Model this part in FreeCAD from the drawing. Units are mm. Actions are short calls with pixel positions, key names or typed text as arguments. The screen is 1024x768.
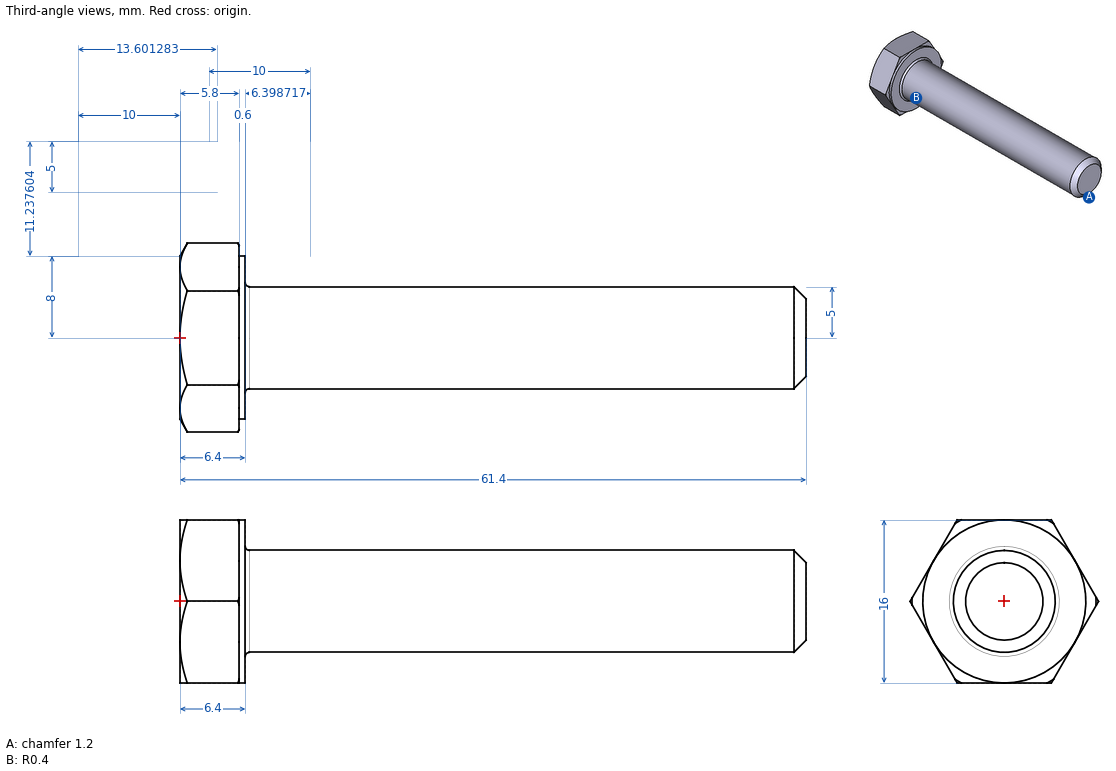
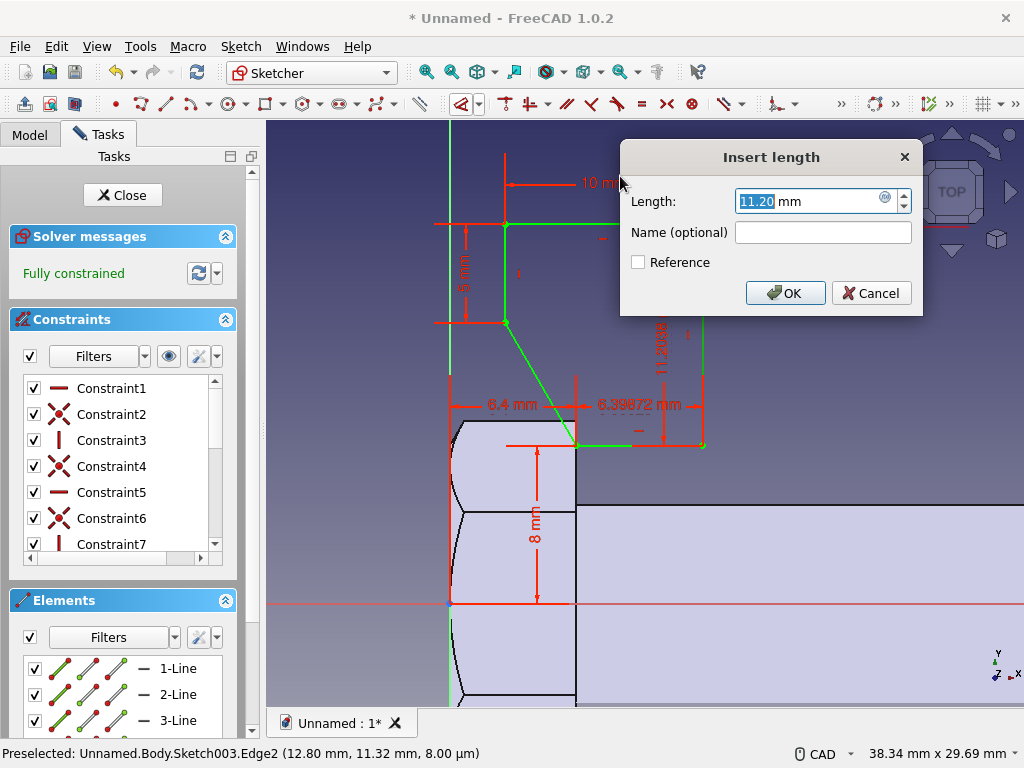
text(11.237604)
key(Return)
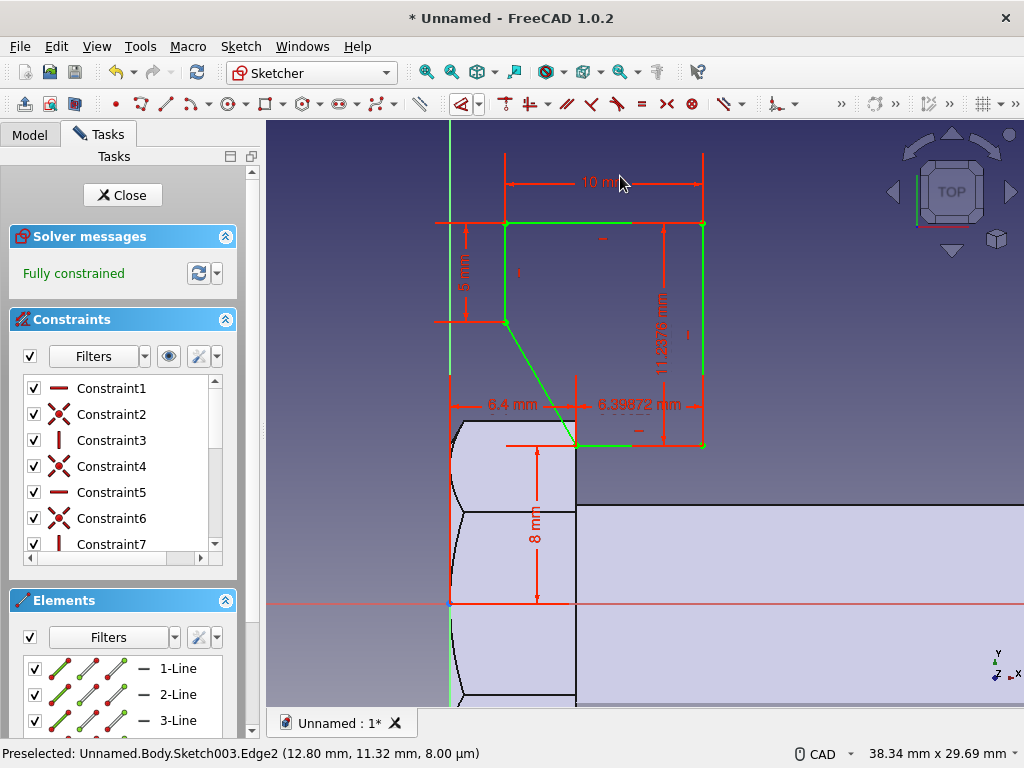
click(123, 195)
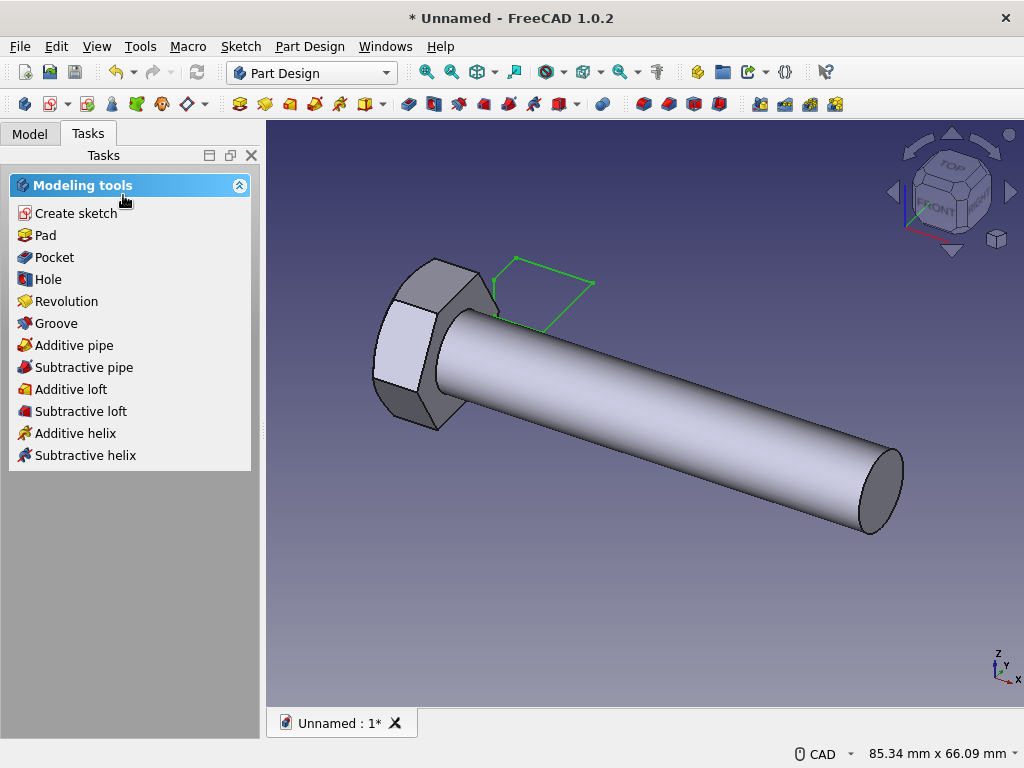
click(459, 104)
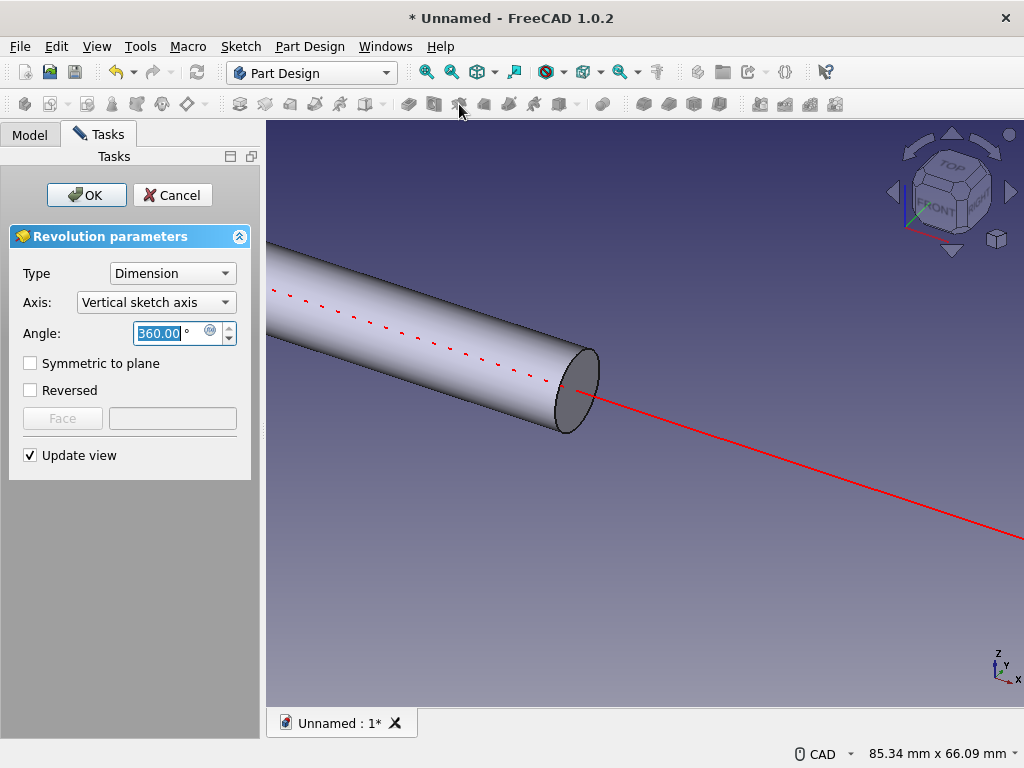
click(157, 302)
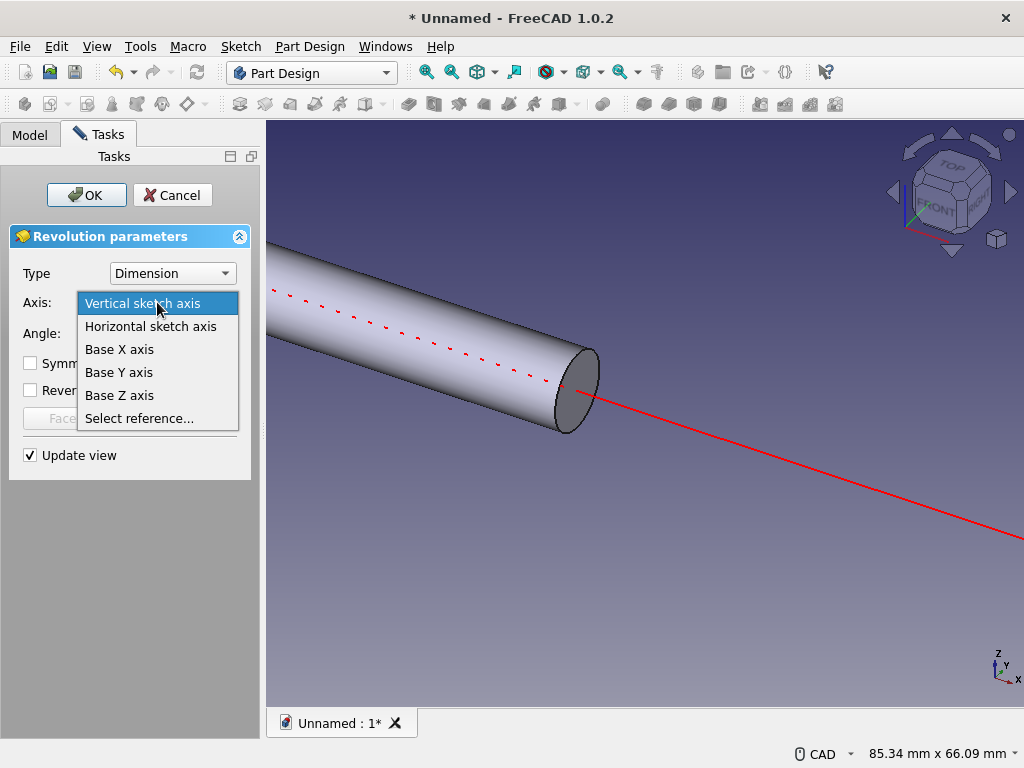
click(156, 326)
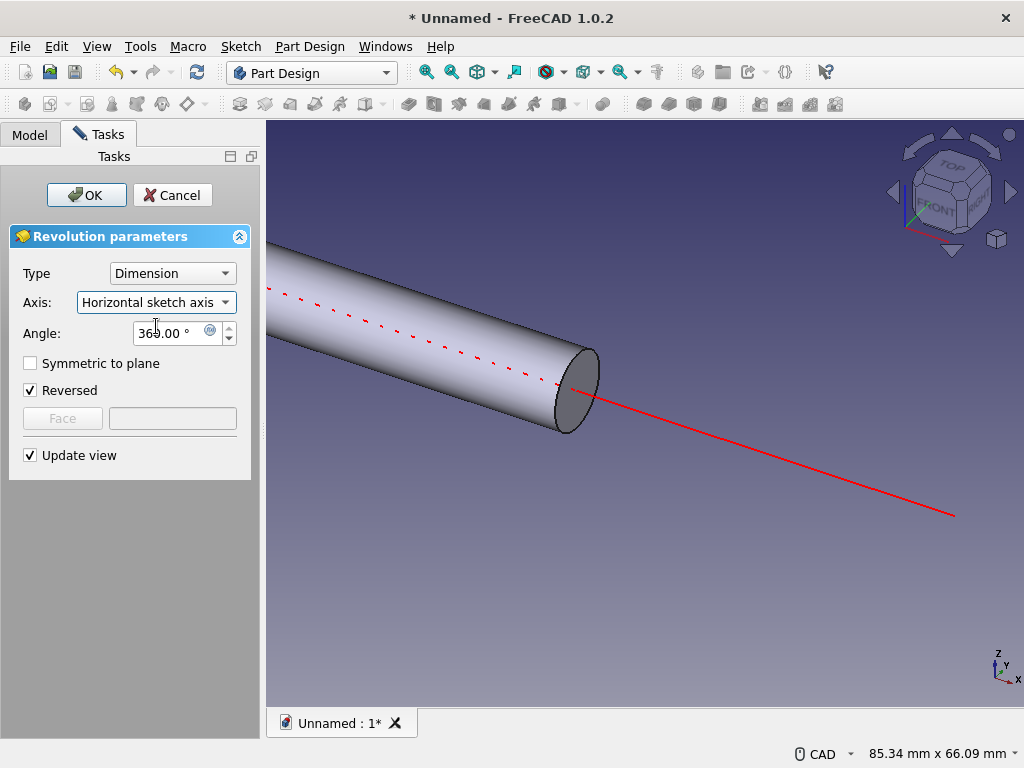
click(87, 195)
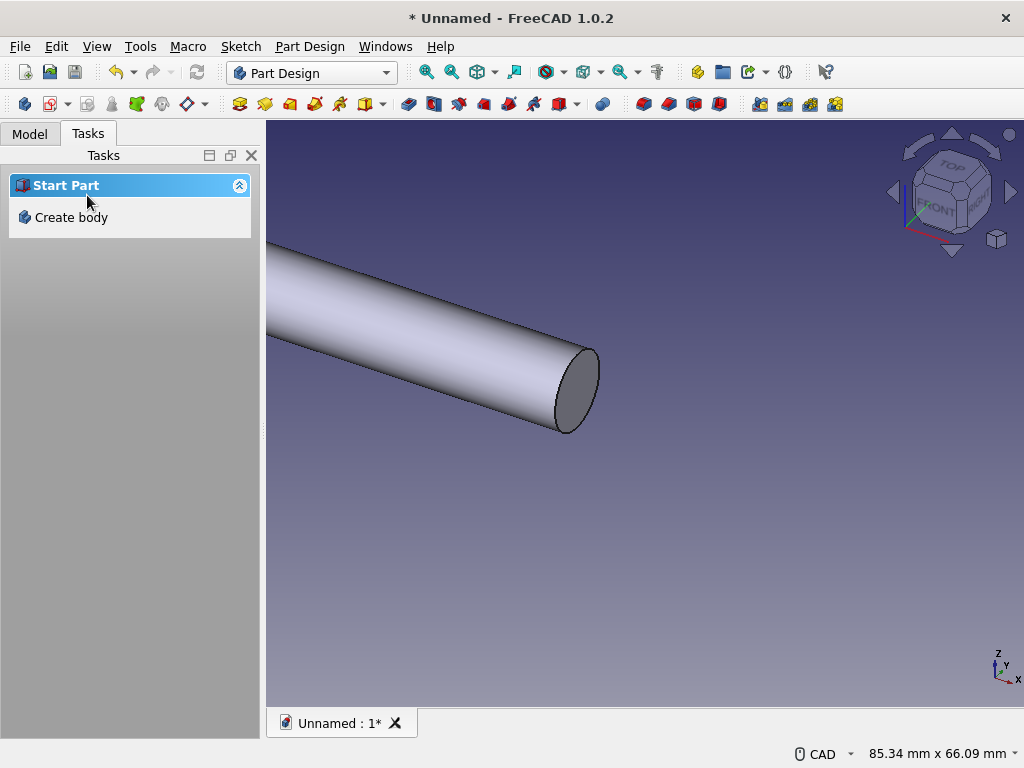
click(427, 72)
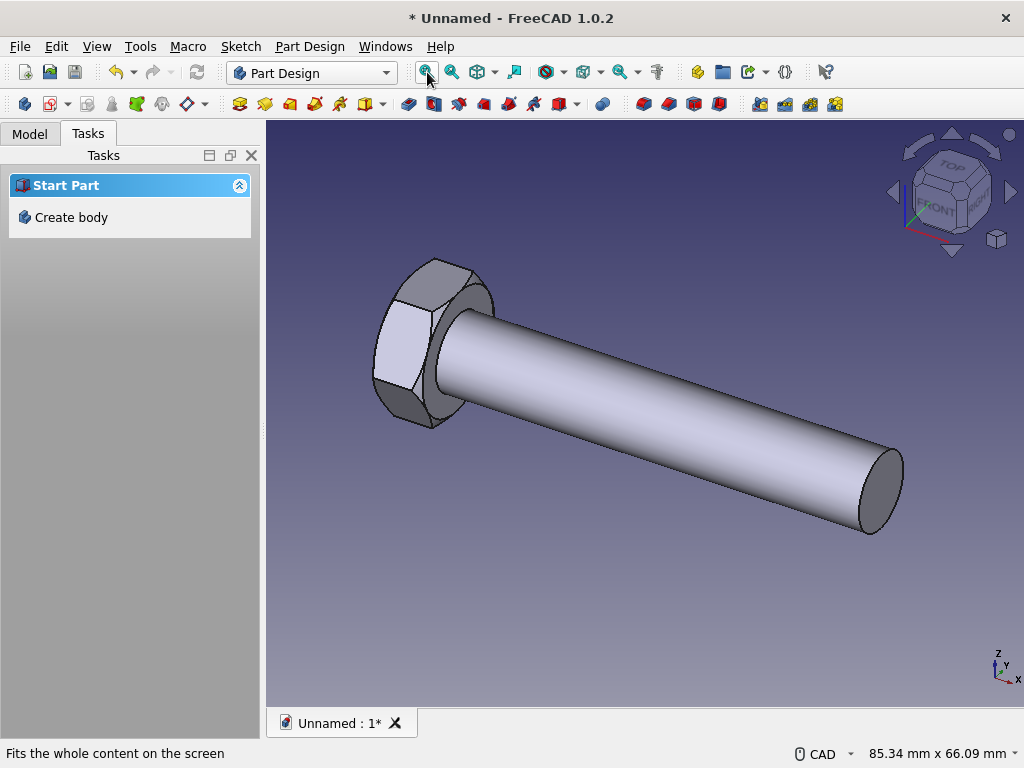
click(50, 104)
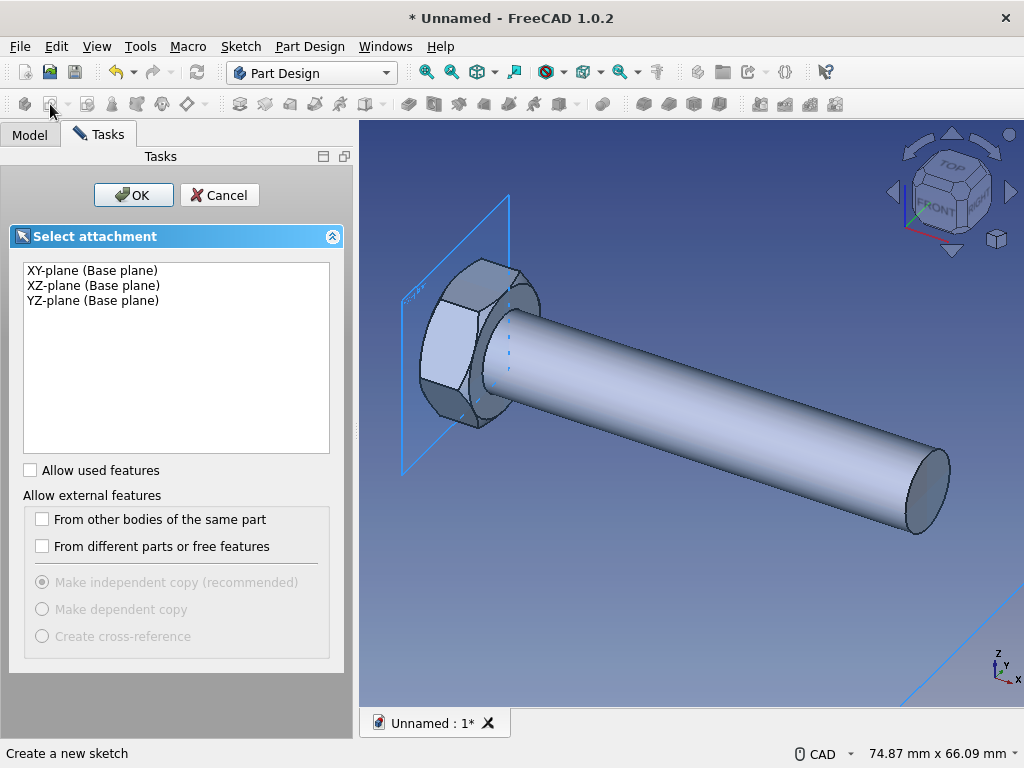
click(84, 270)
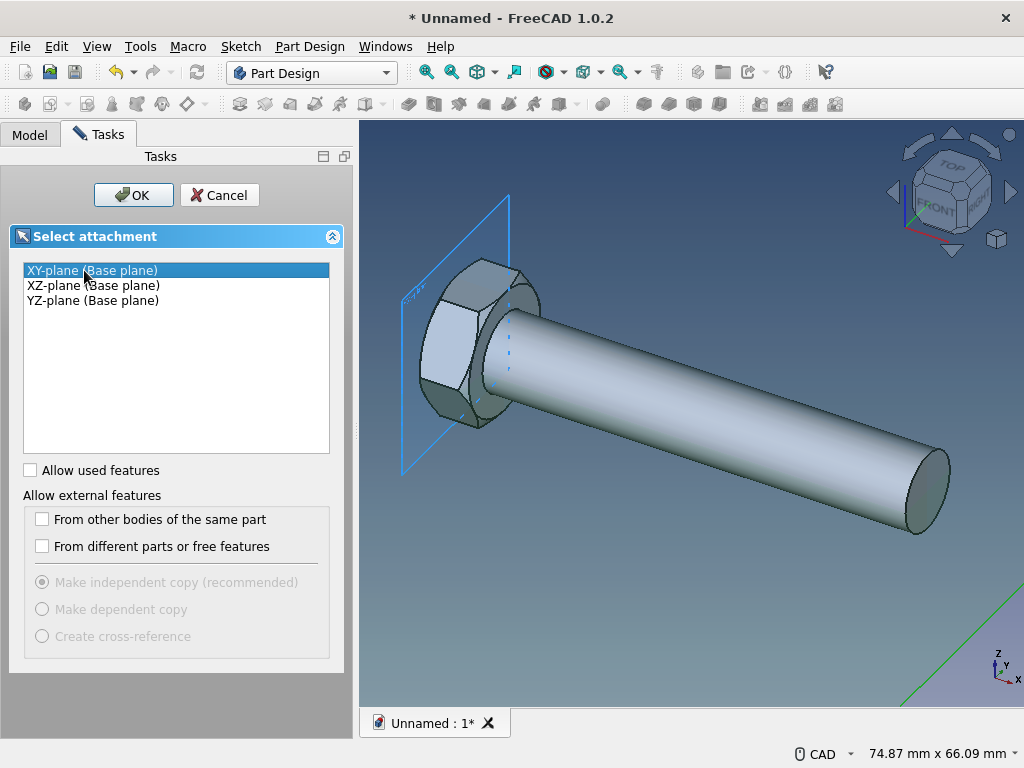
click(134, 195)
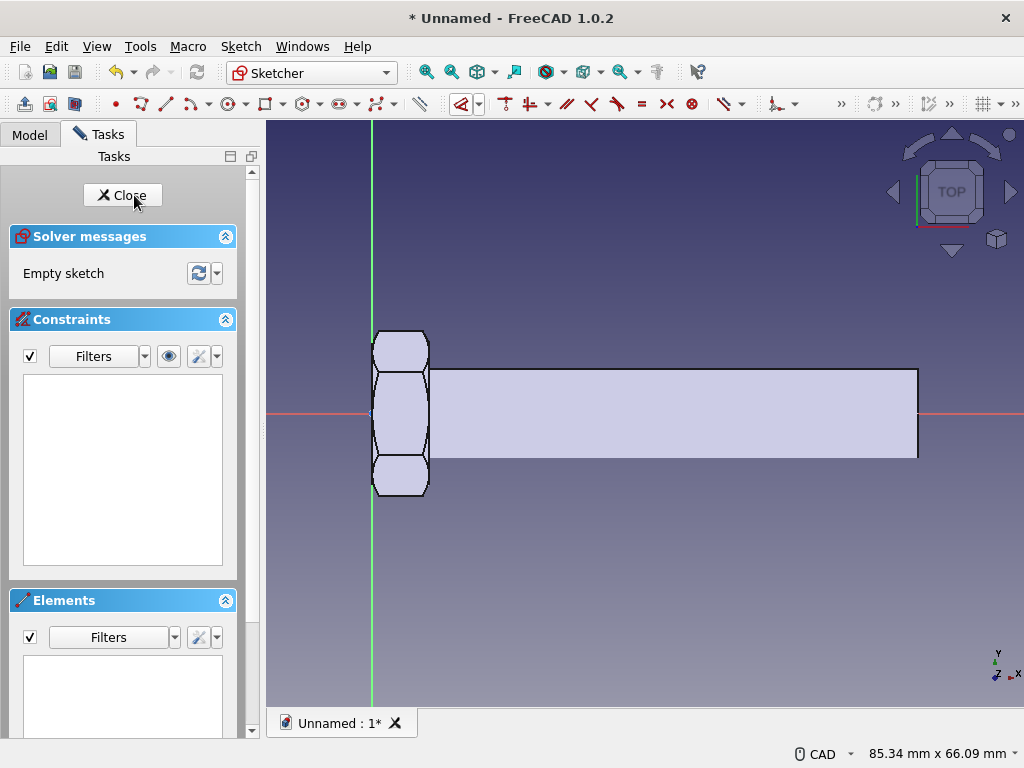
click(75, 104)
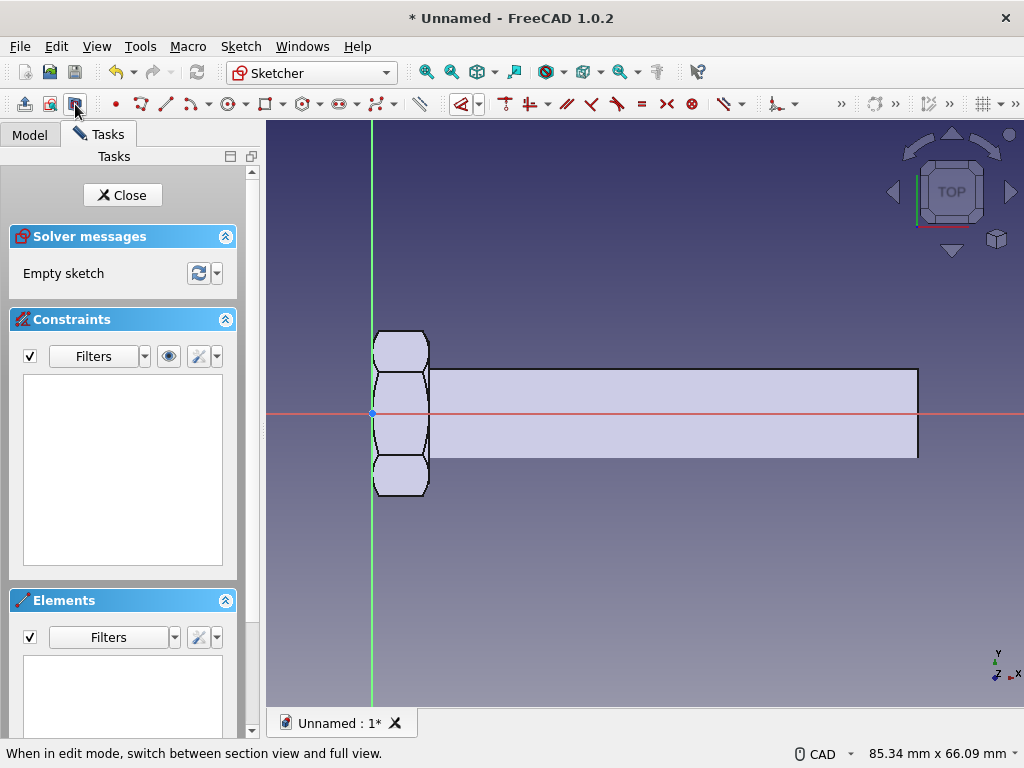
scroll(294, 258, up, 4)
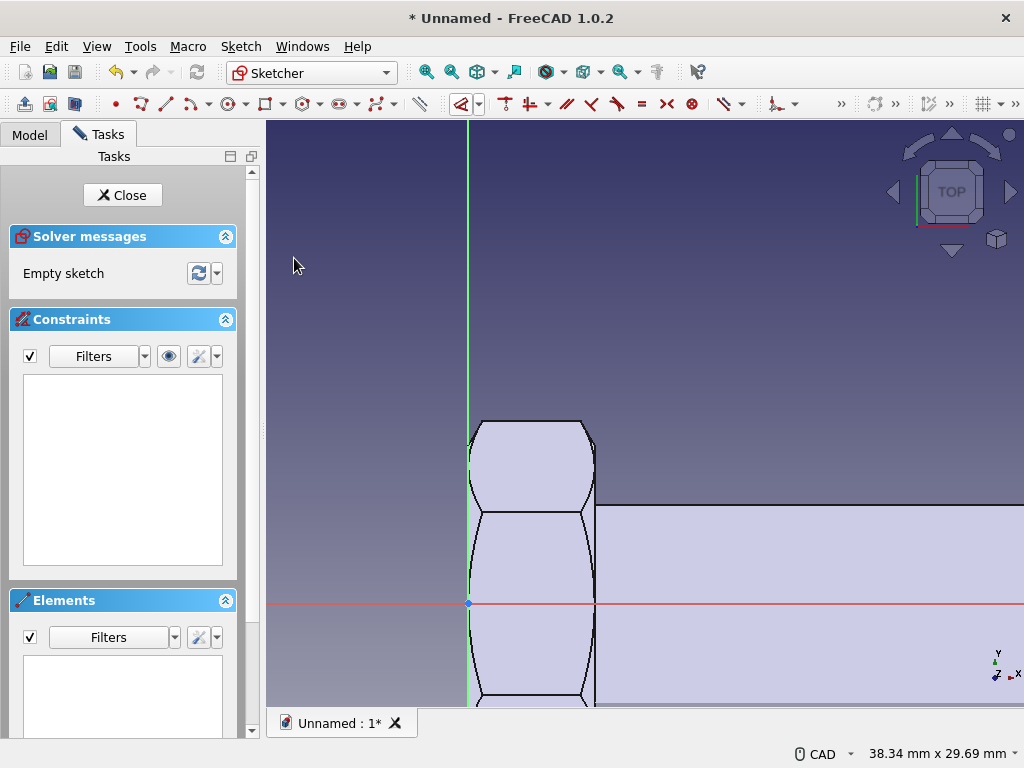
click(264, 104)